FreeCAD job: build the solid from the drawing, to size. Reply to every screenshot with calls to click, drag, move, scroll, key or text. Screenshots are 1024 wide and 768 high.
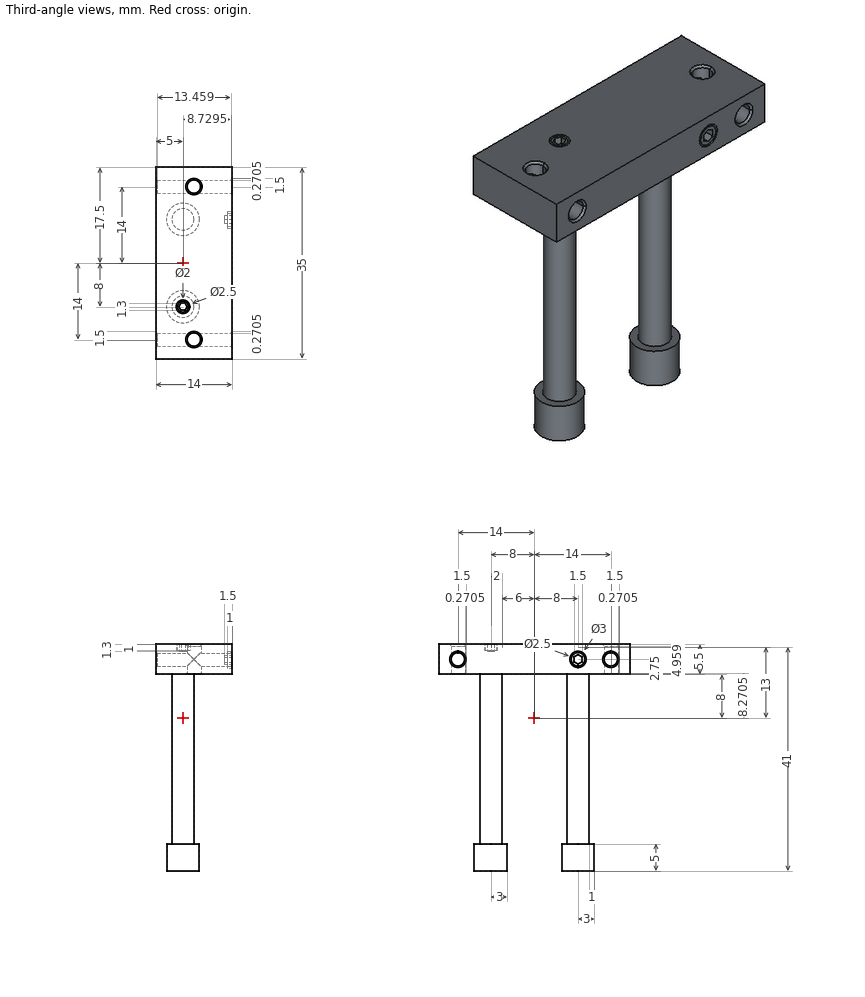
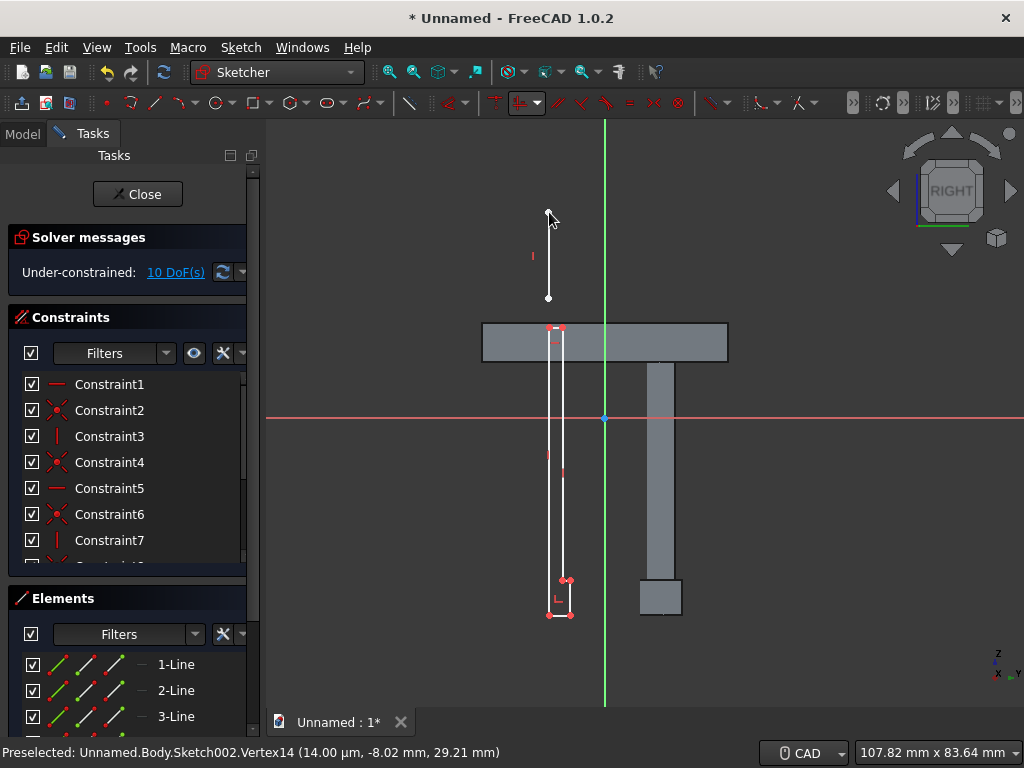
click(549, 273)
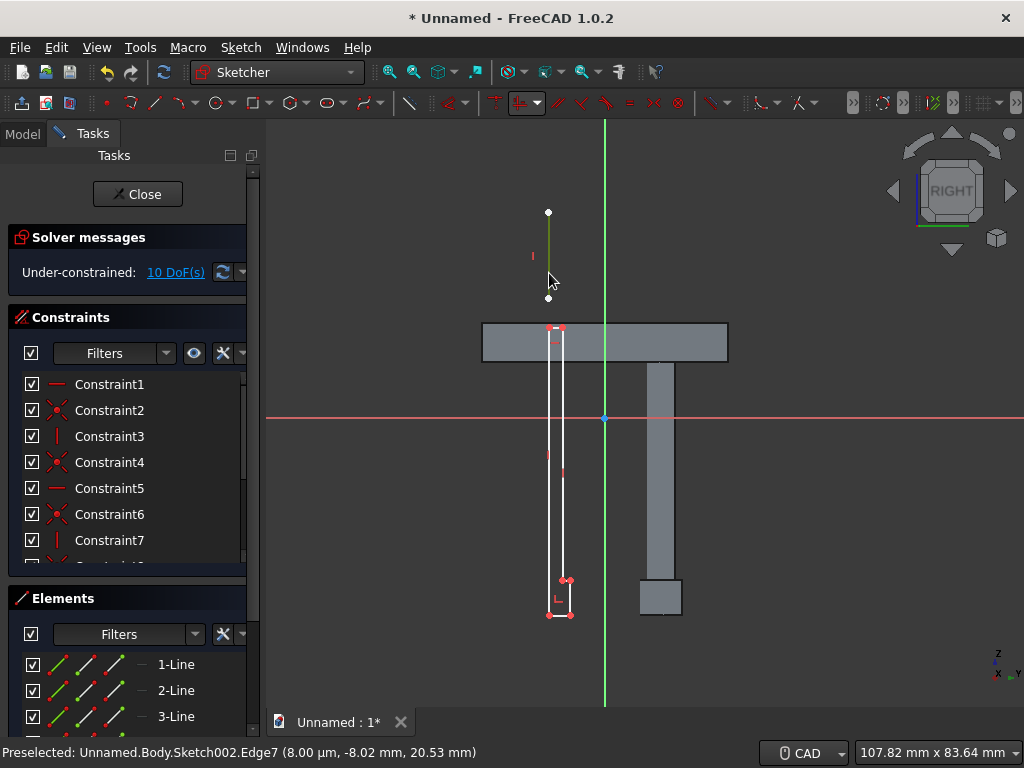
click(410, 104)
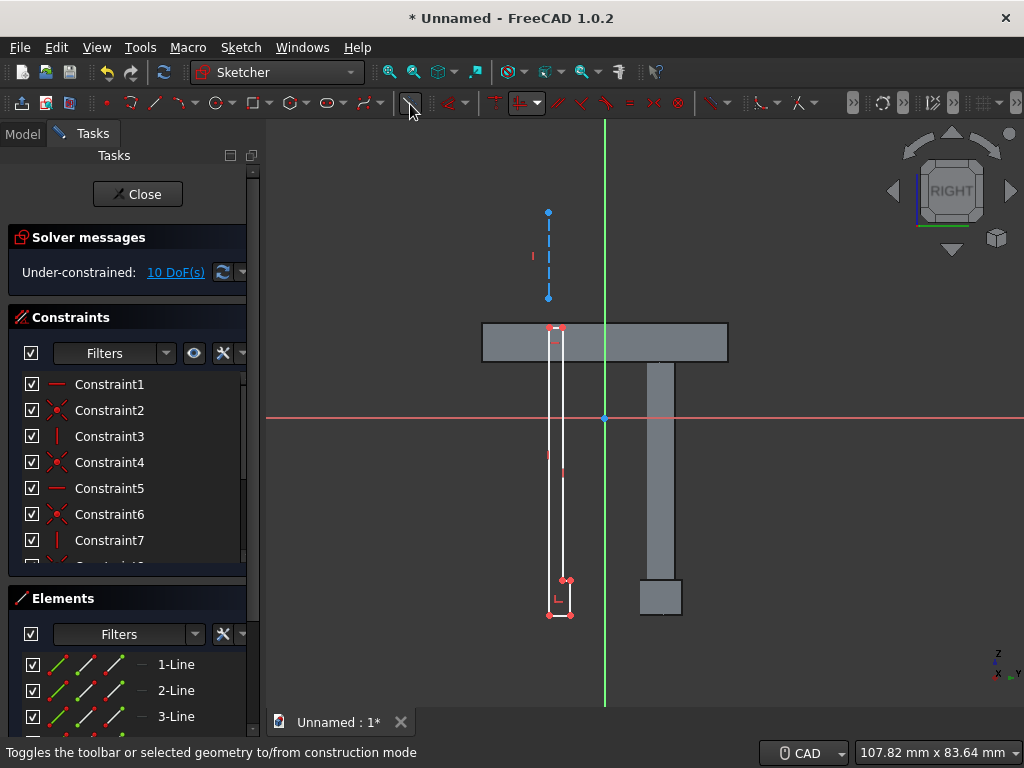
scroll(566, 581, up, 7)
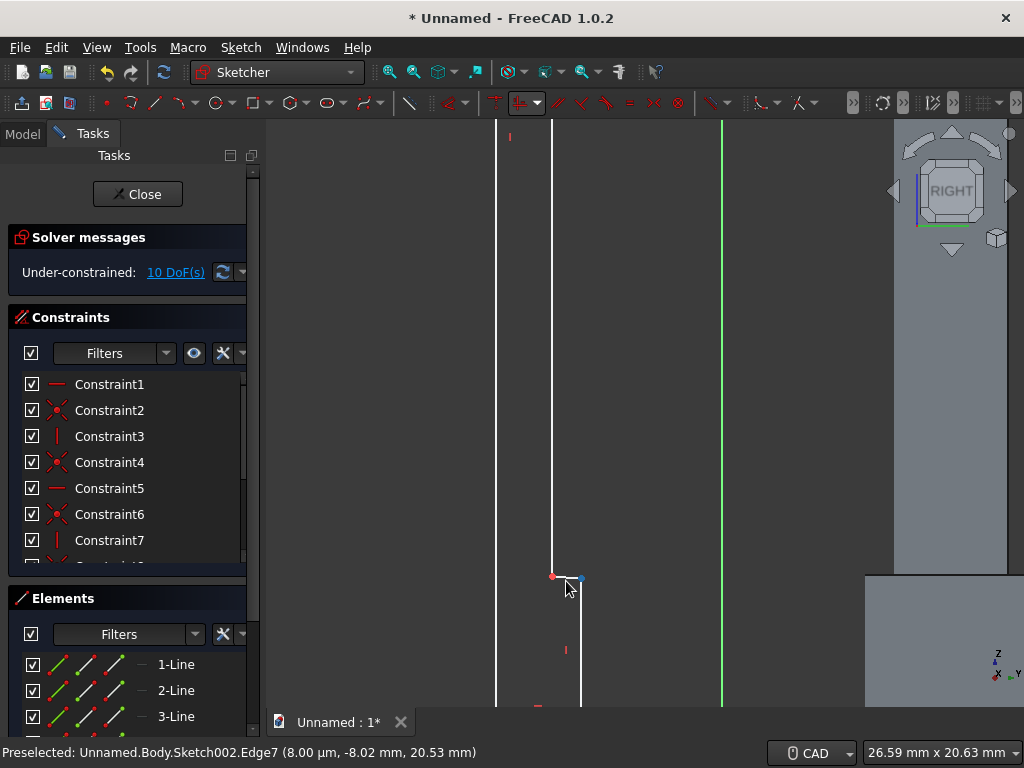
click(567, 578)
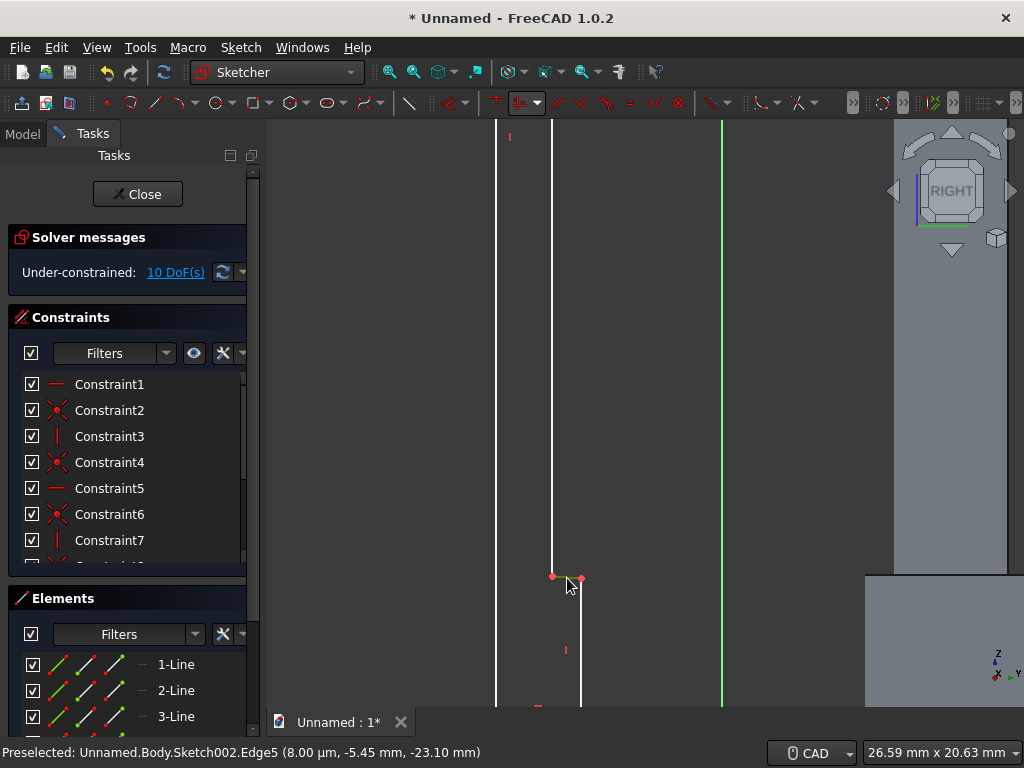
click(540, 104)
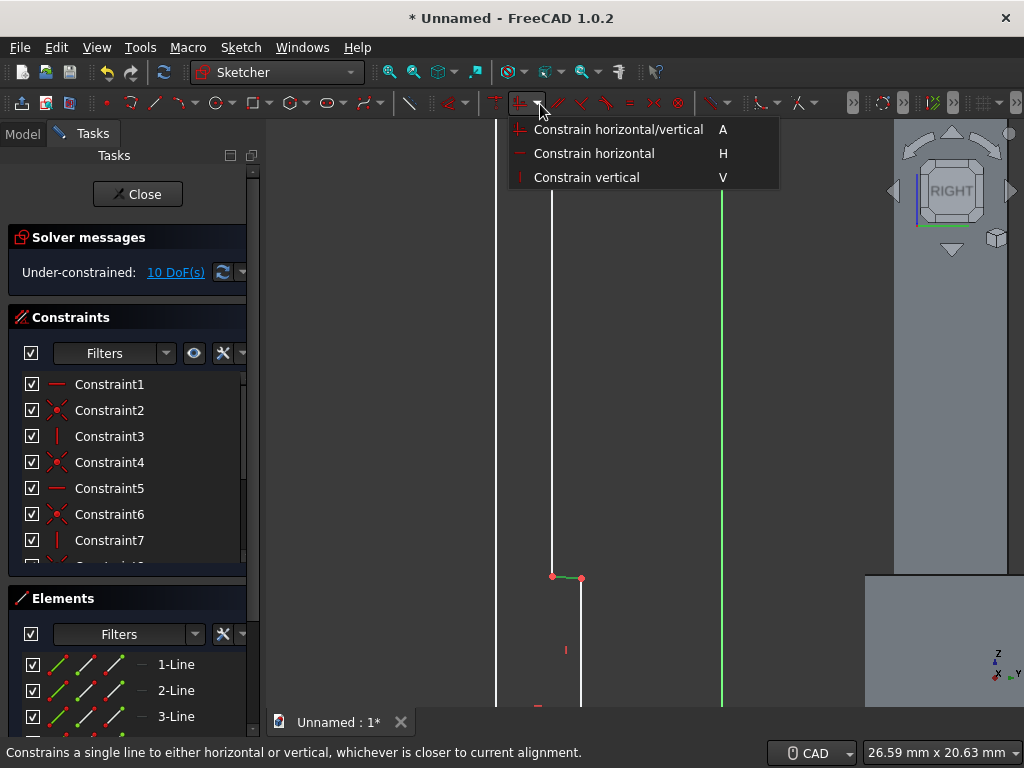
click(644, 153)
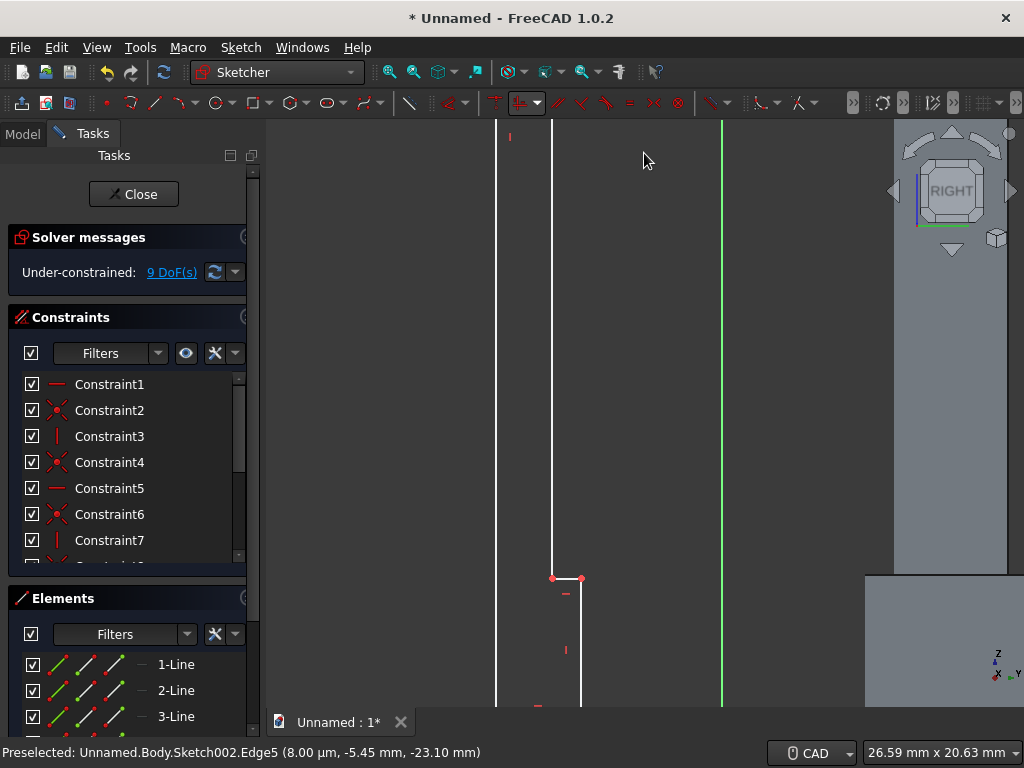
click(448, 104)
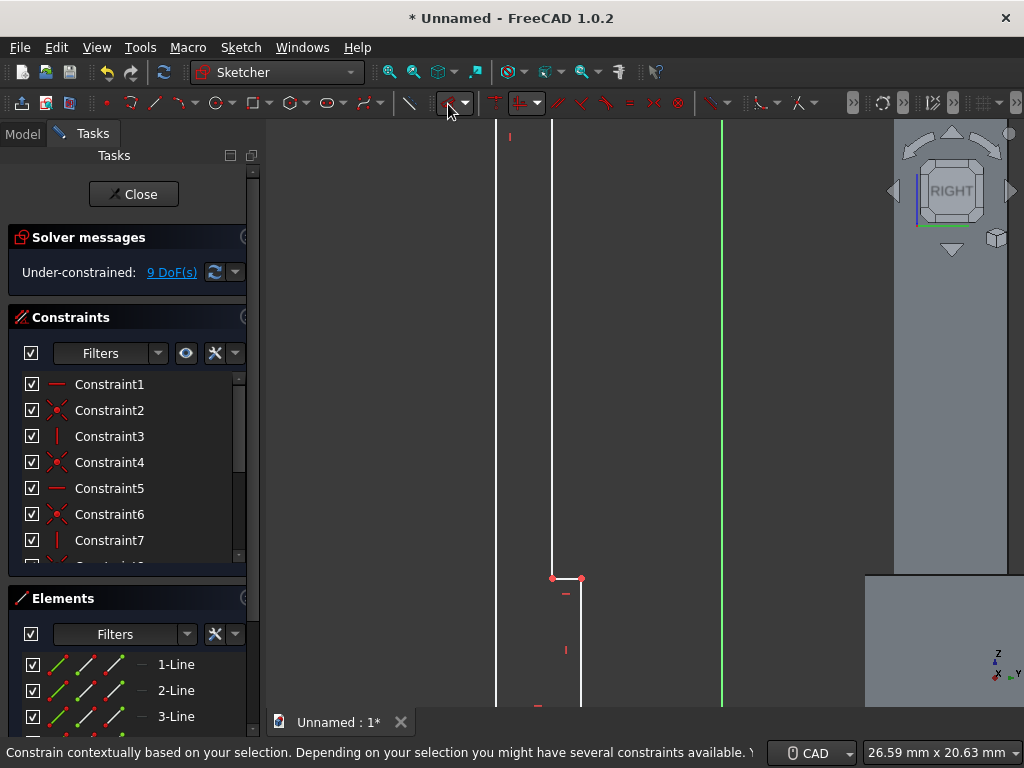
scroll(566, 581, down, 7)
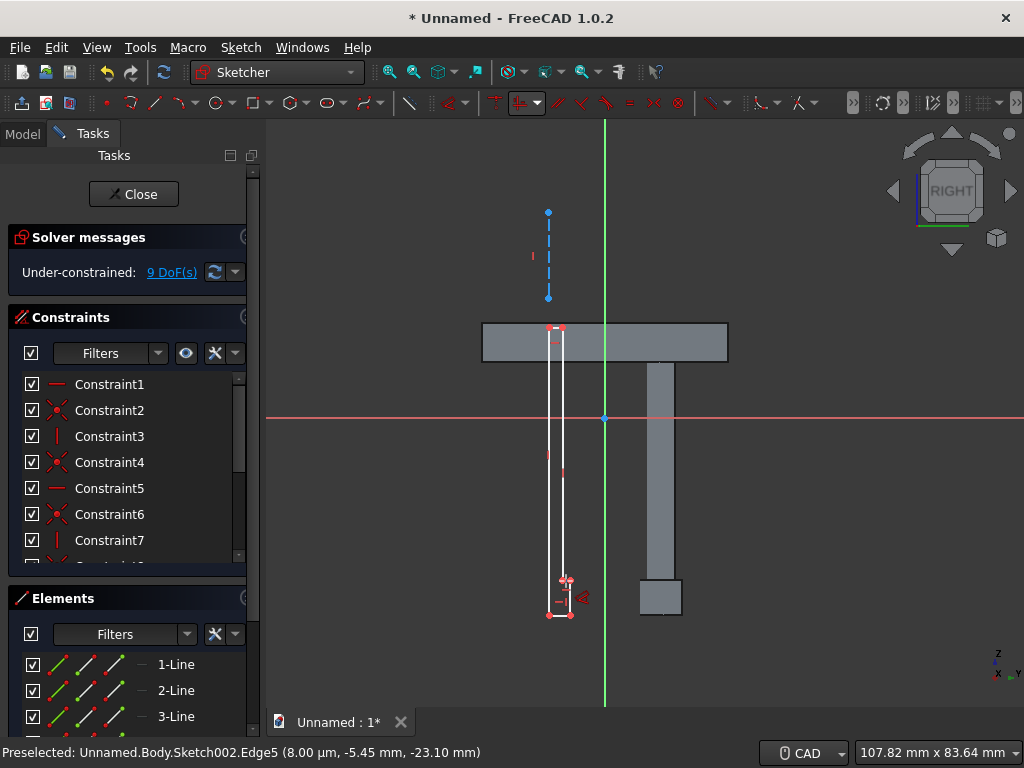
scroll(559, 328, up, 6)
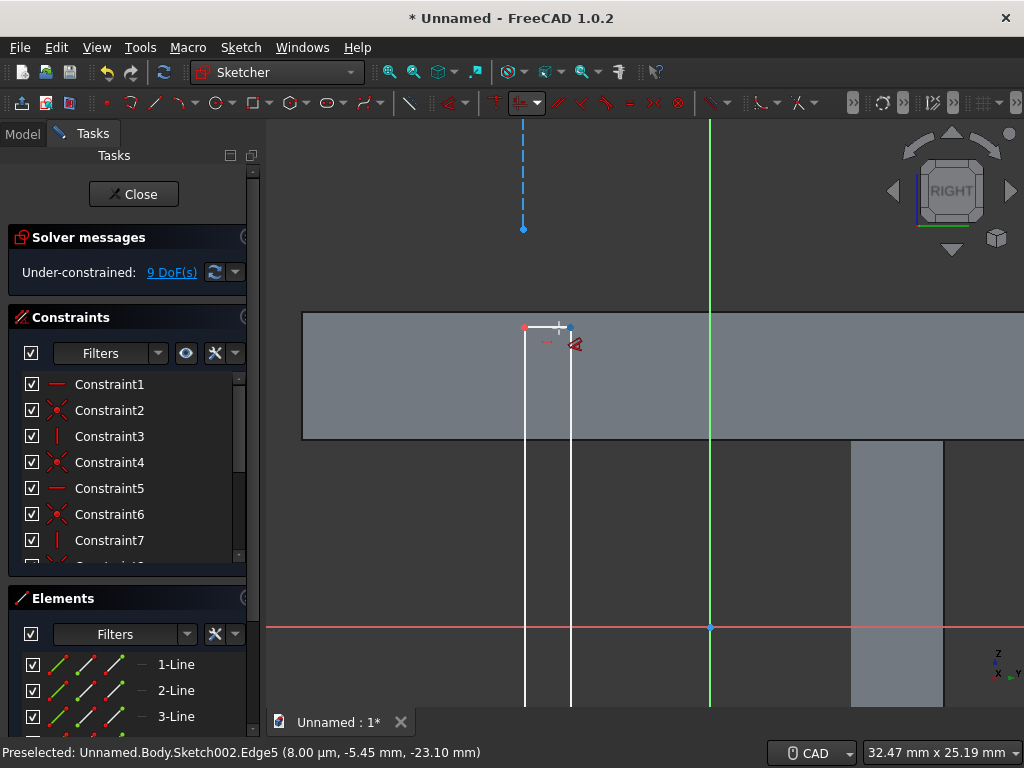
click(557, 327)
click(548, 293)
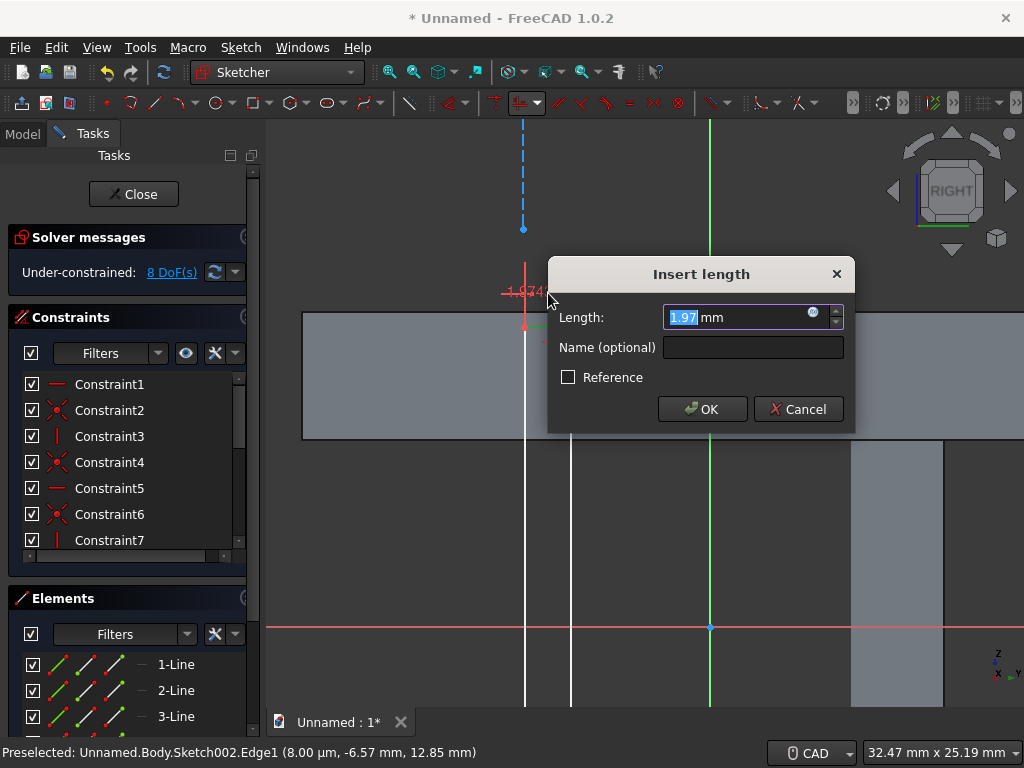
text(2)
key(Return)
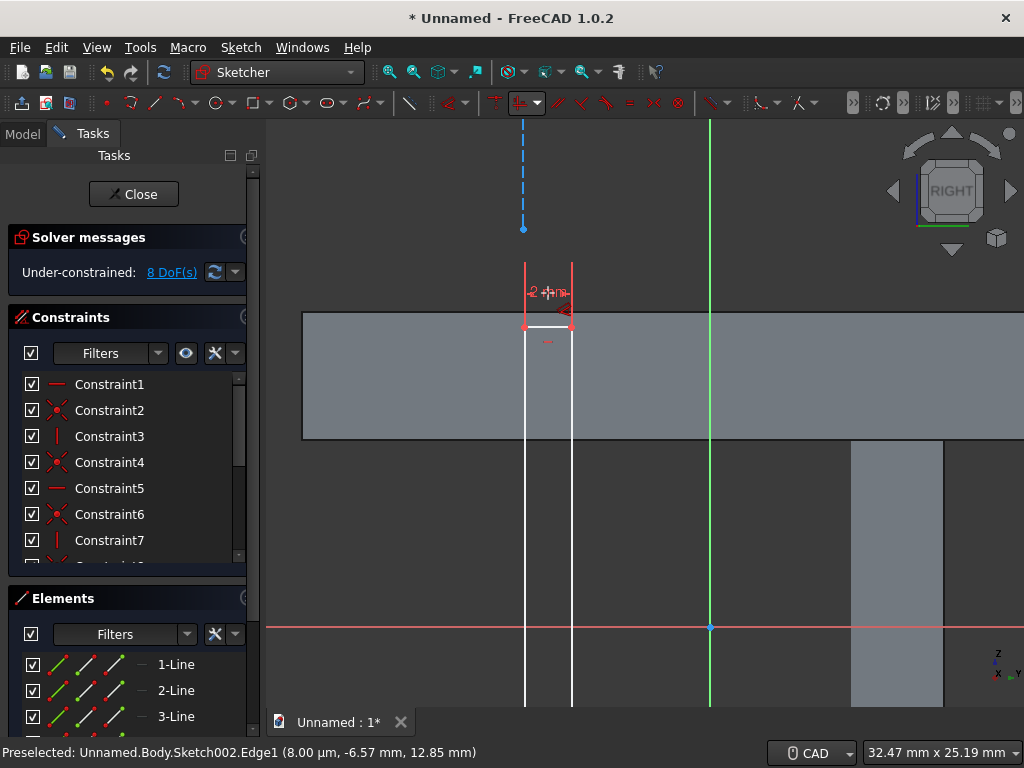
scroll(559, 328, down, 6)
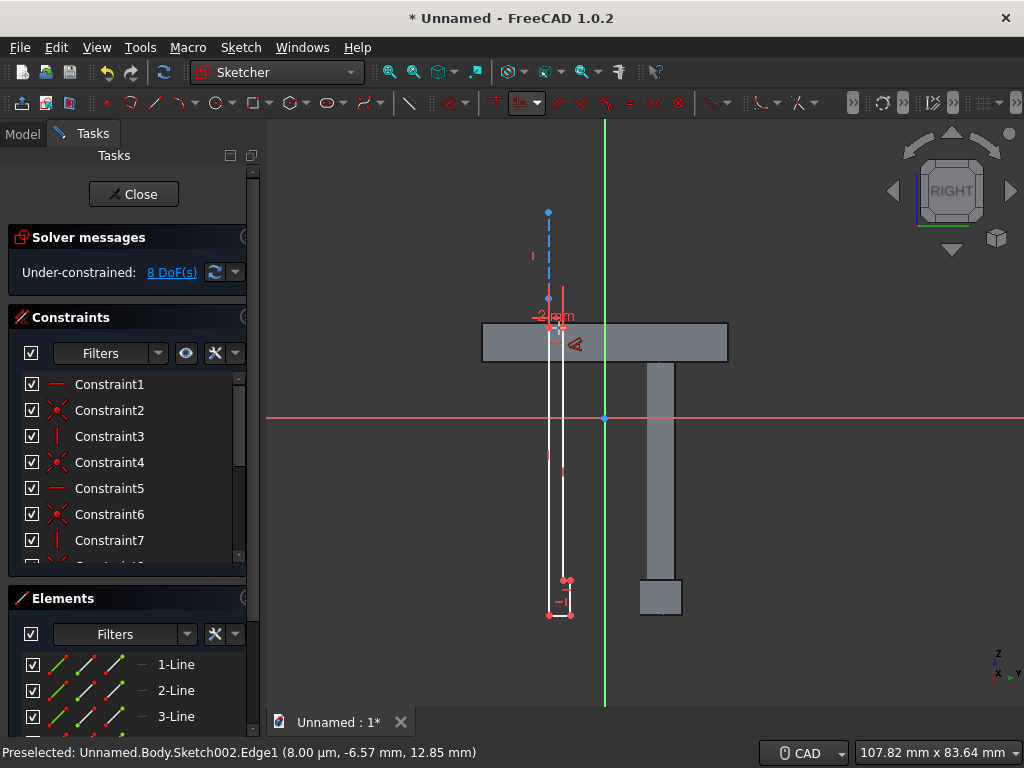
scroll(555, 616, up, 4)